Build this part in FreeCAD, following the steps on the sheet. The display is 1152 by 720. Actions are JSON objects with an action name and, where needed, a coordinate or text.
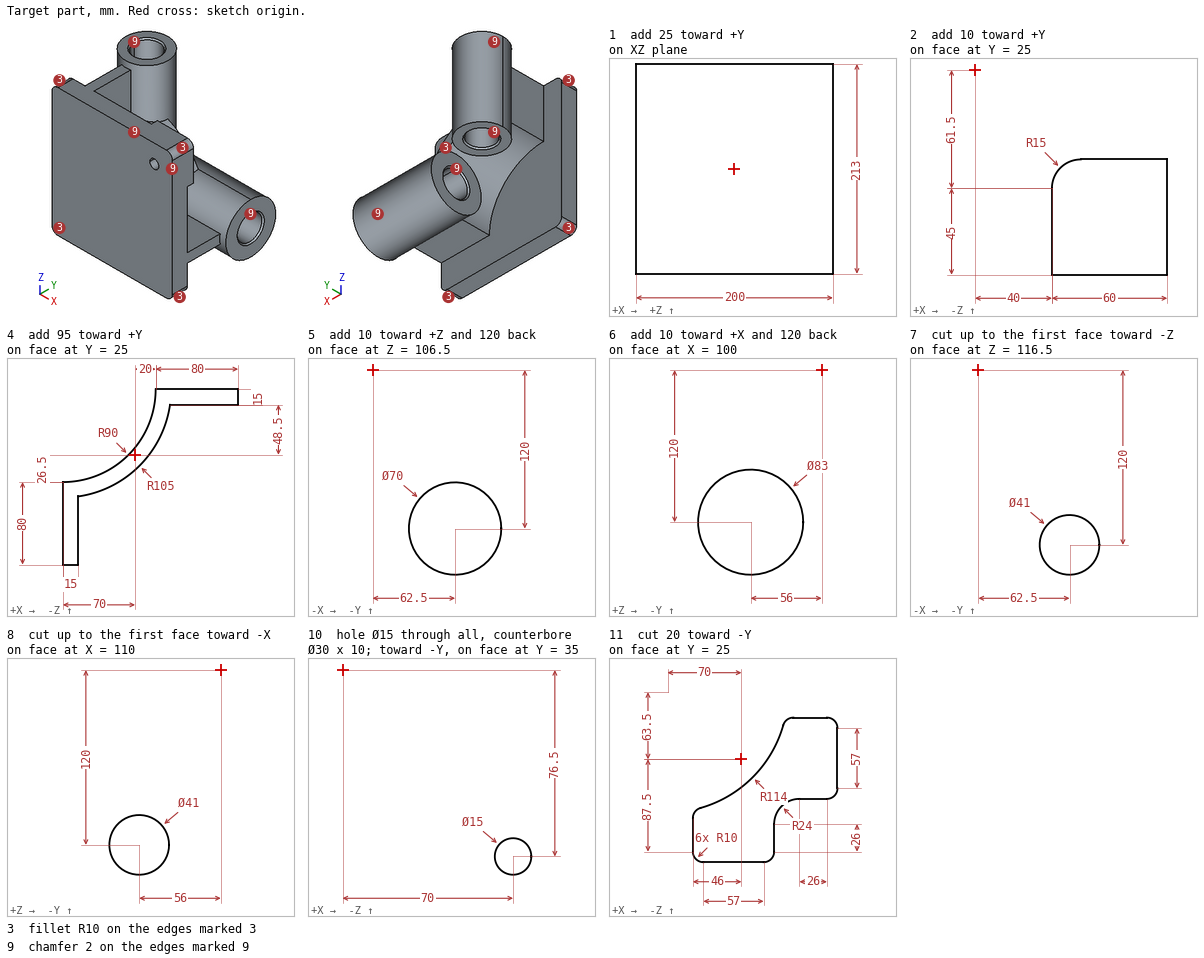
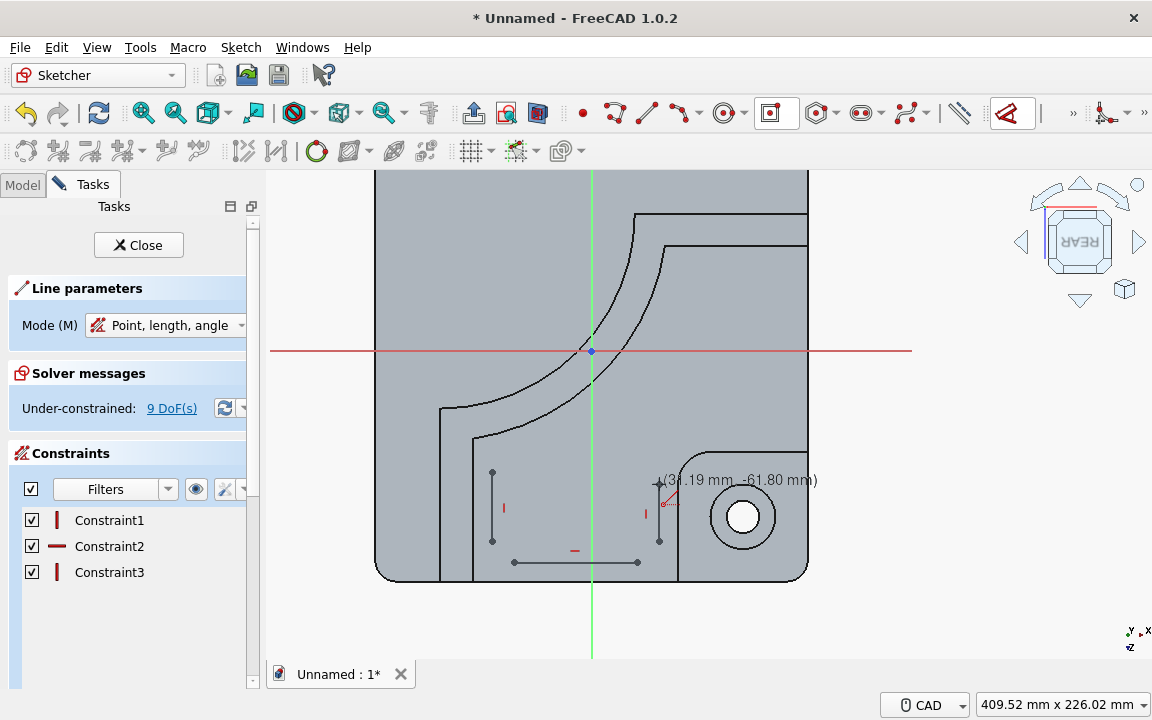
{"action": "left_click", "coordinate": [711, 432]}
{"action": "left_click", "coordinate": [767, 432]}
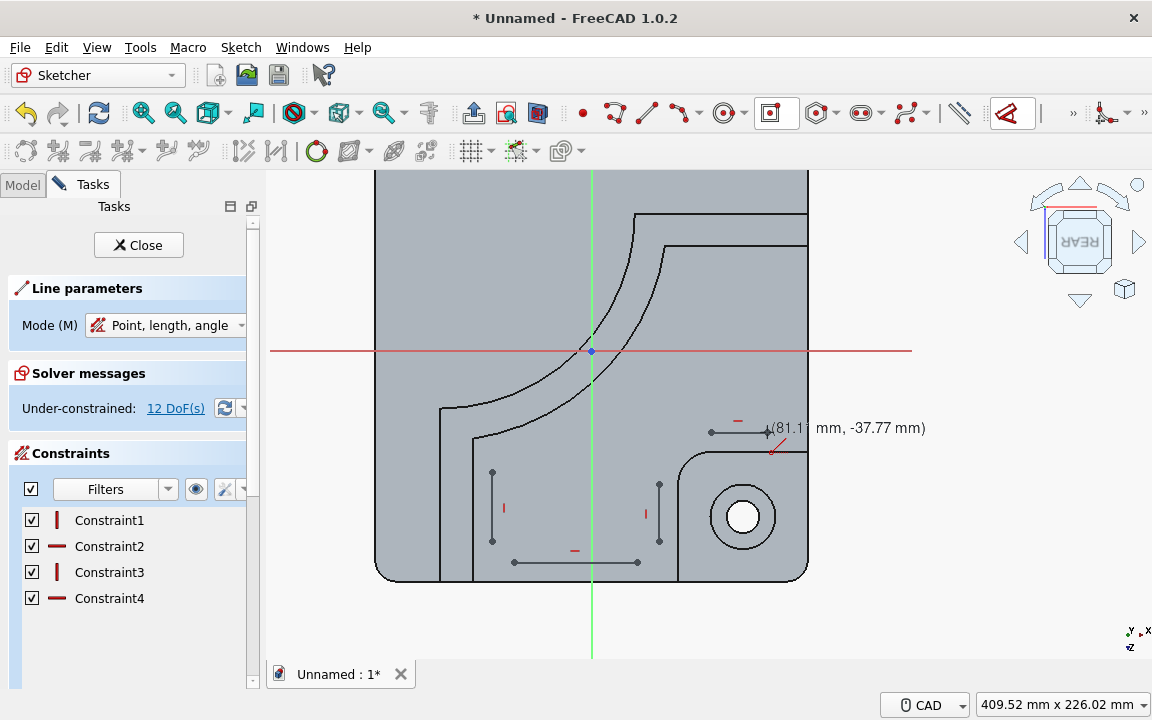
{"action": "left_click", "coordinate": [788, 411]}
{"action": "left_click", "coordinate": [788, 287]}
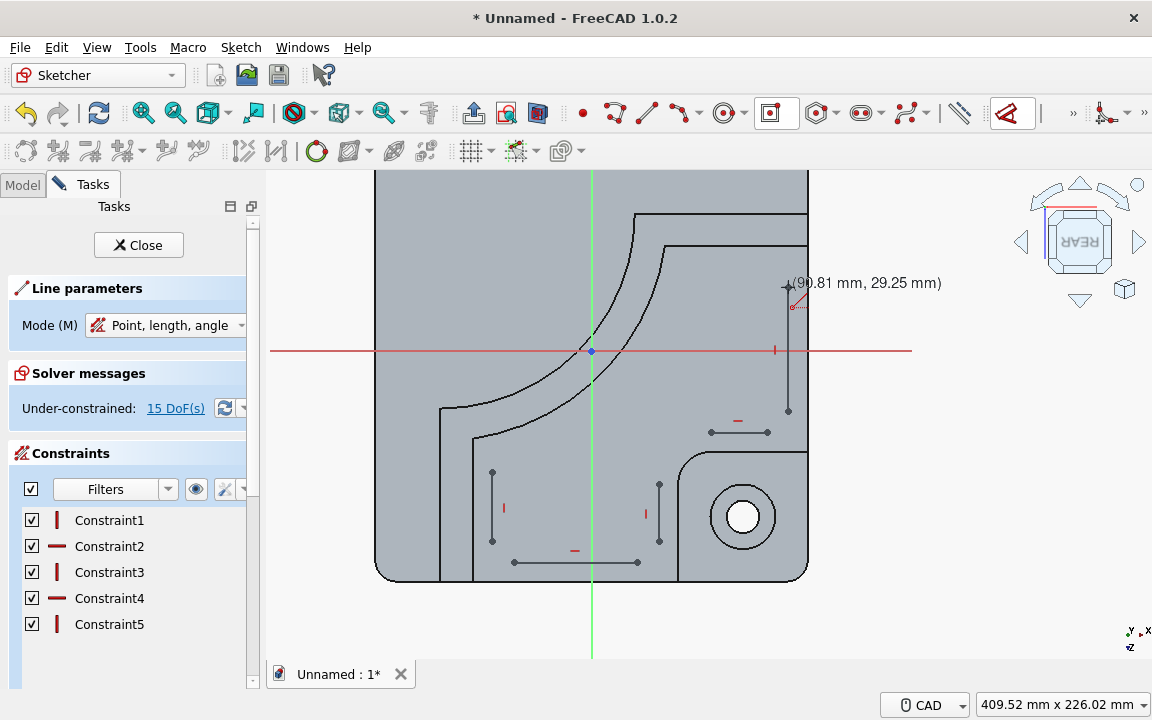
{"action": "left_click", "coordinate": [767, 266]}
{"action": "left_click", "coordinate": [698, 266]}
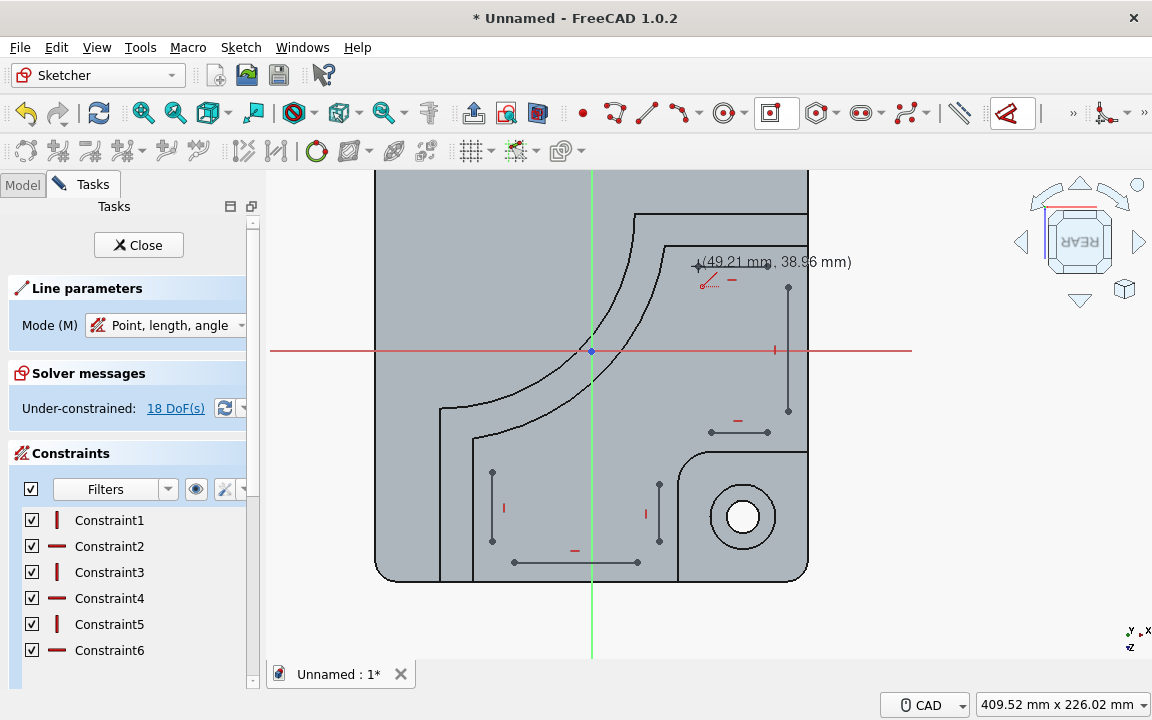
{"action": "left_click", "coordinate": [680, 114]}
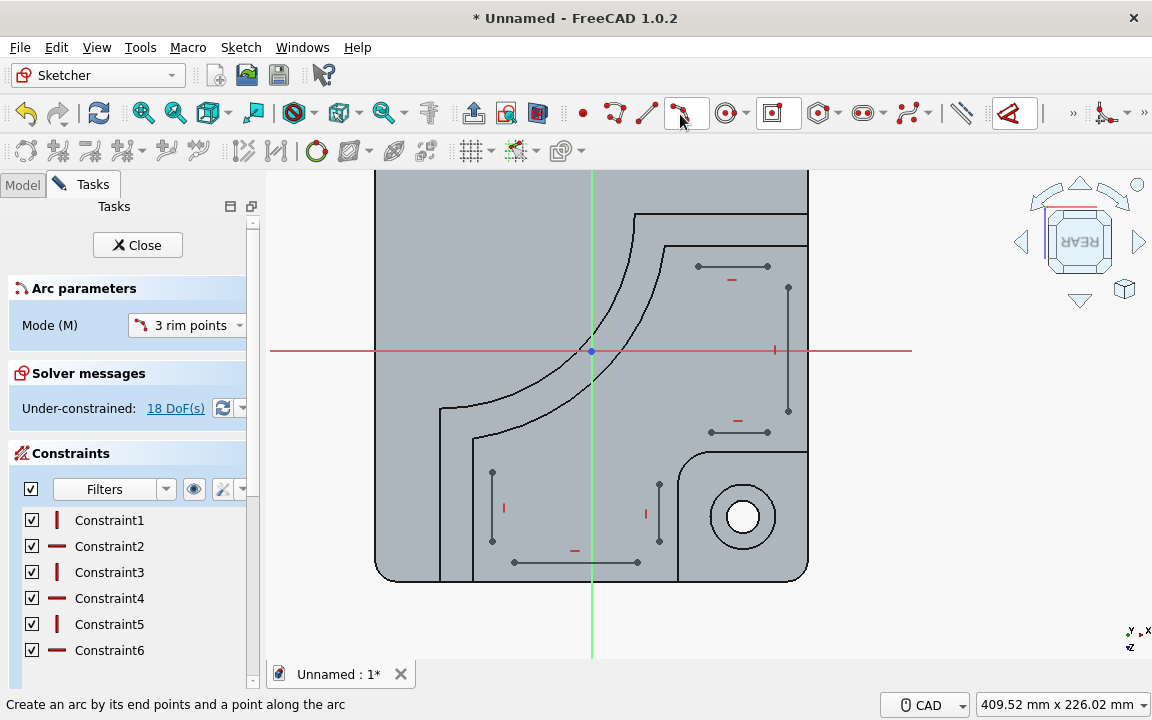
{"action": "left_click", "coordinate": [492, 542]}
{"action": "left_click", "coordinate": [514, 563]}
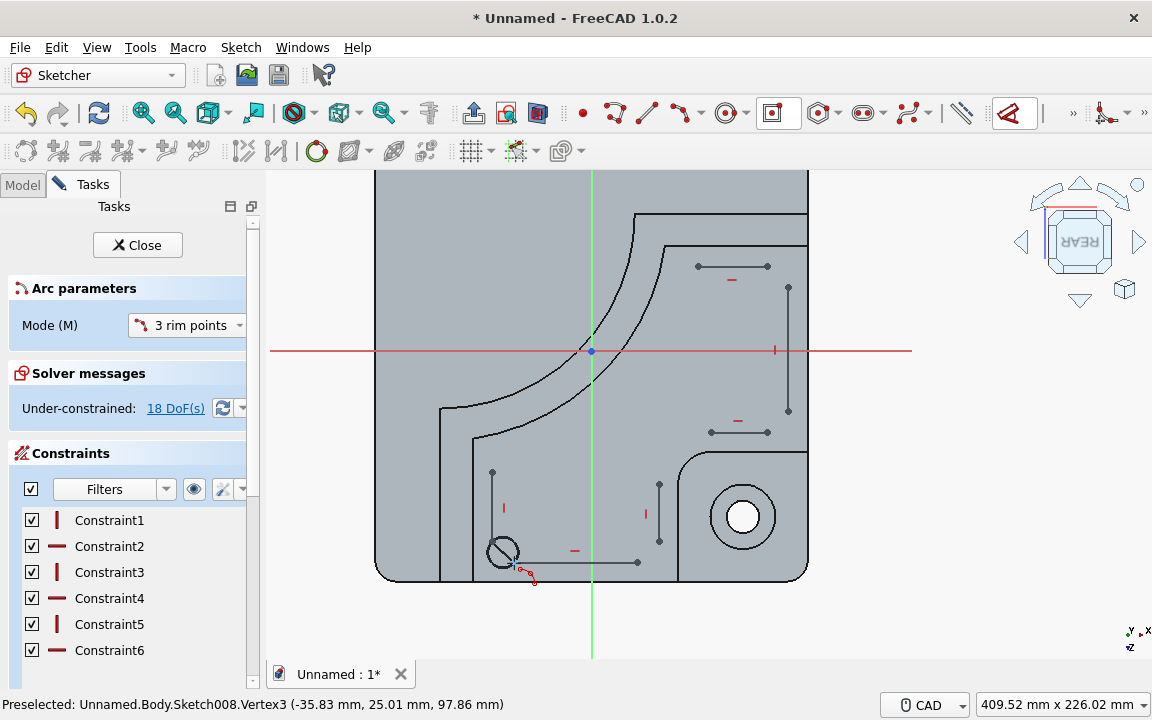
{"action": "scroll", "coordinate": [498, 556], "scroll_direction": "up", "scroll_amount": 5}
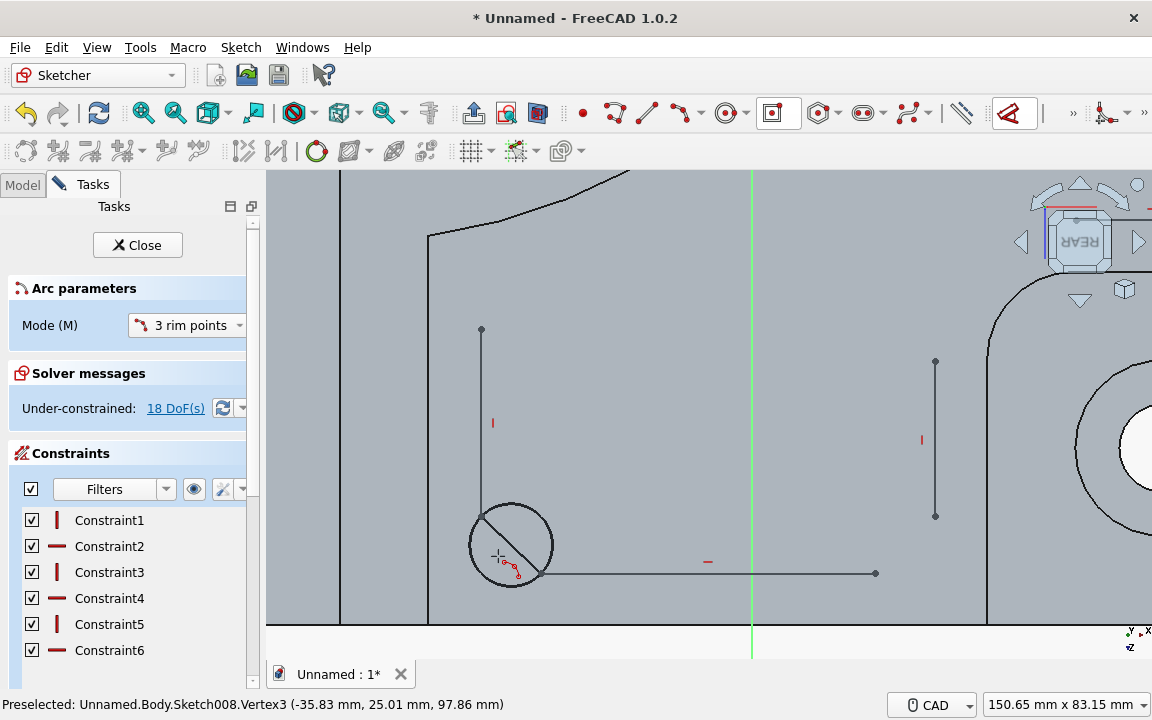
{"action": "left_click", "coordinate": [498, 554]}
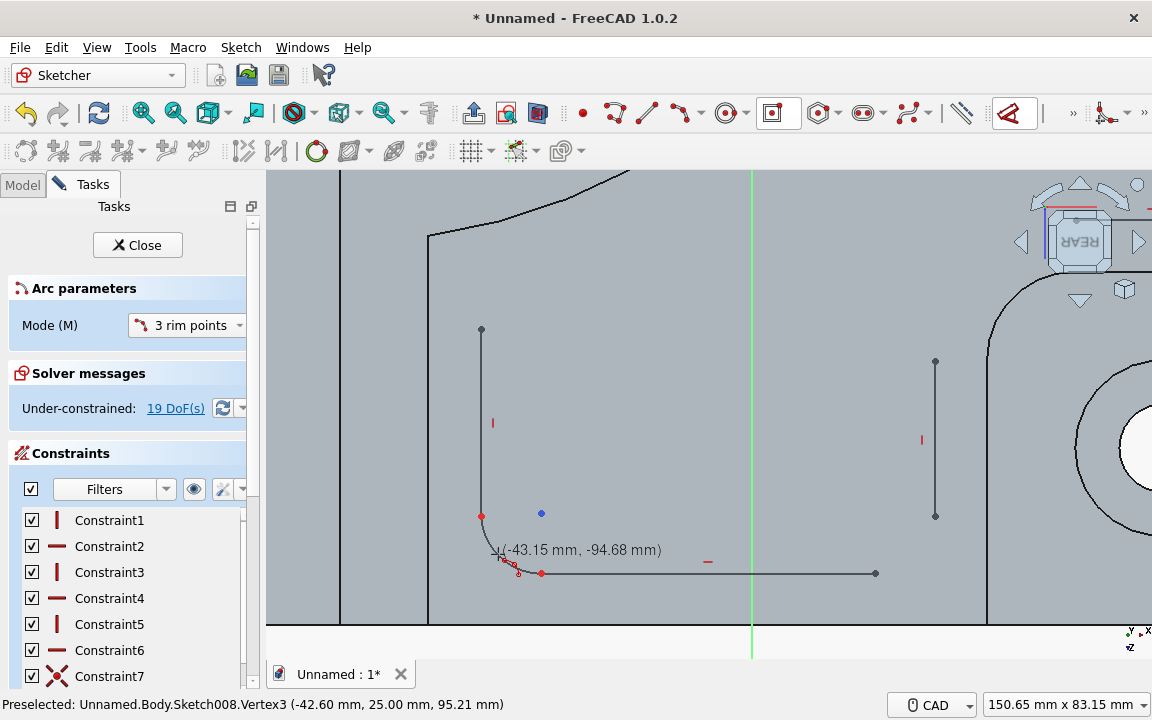
{"action": "left_click", "coordinate": [875, 574]}
{"action": "left_click", "coordinate": [935, 517]}
{"action": "left_click", "coordinate": [917, 554]}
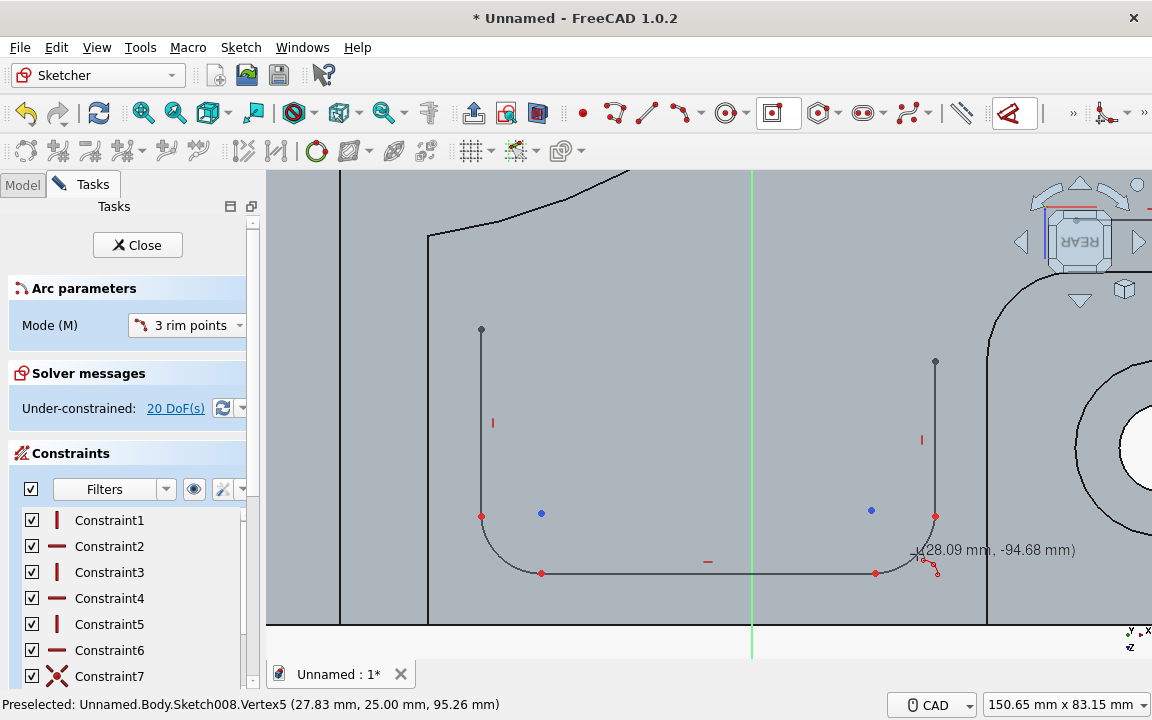
{"action": "left_click", "coordinate": [935, 362]}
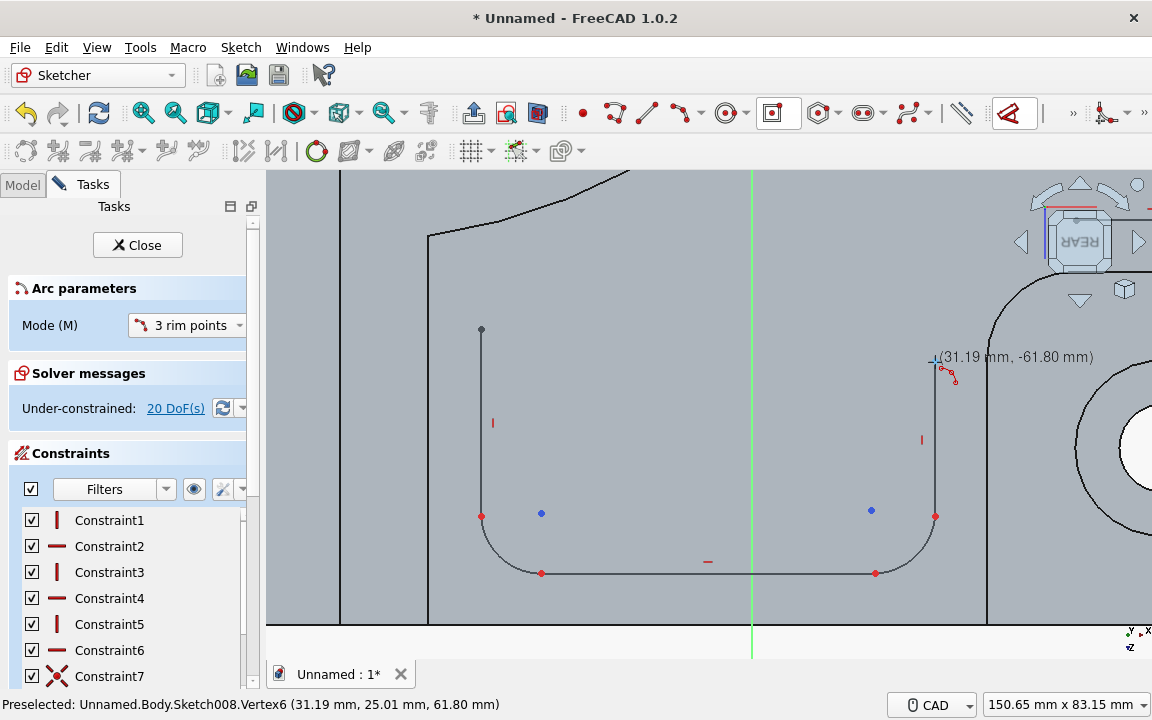
{"action": "scroll", "coordinate": [499, 558], "scroll_direction": "down", "scroll_amount": 5}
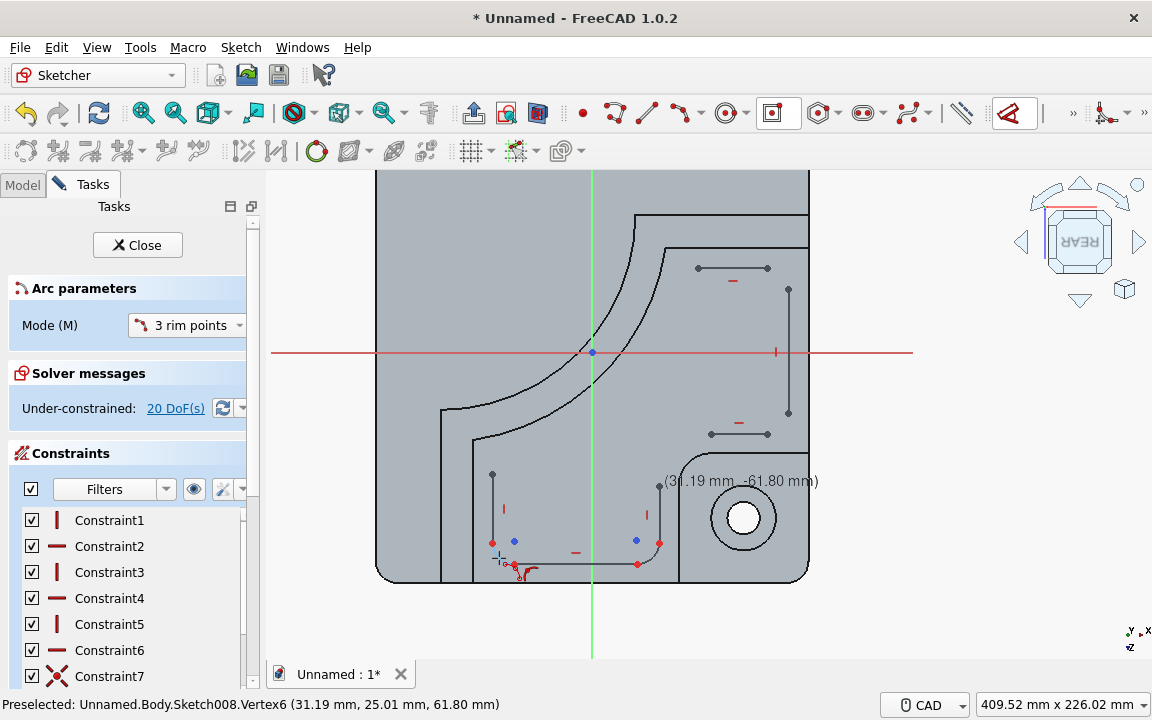
{"action": "left_click", "coordinate": [712, 434]}
{"action": "left_click", "coordinate": [674, 449]}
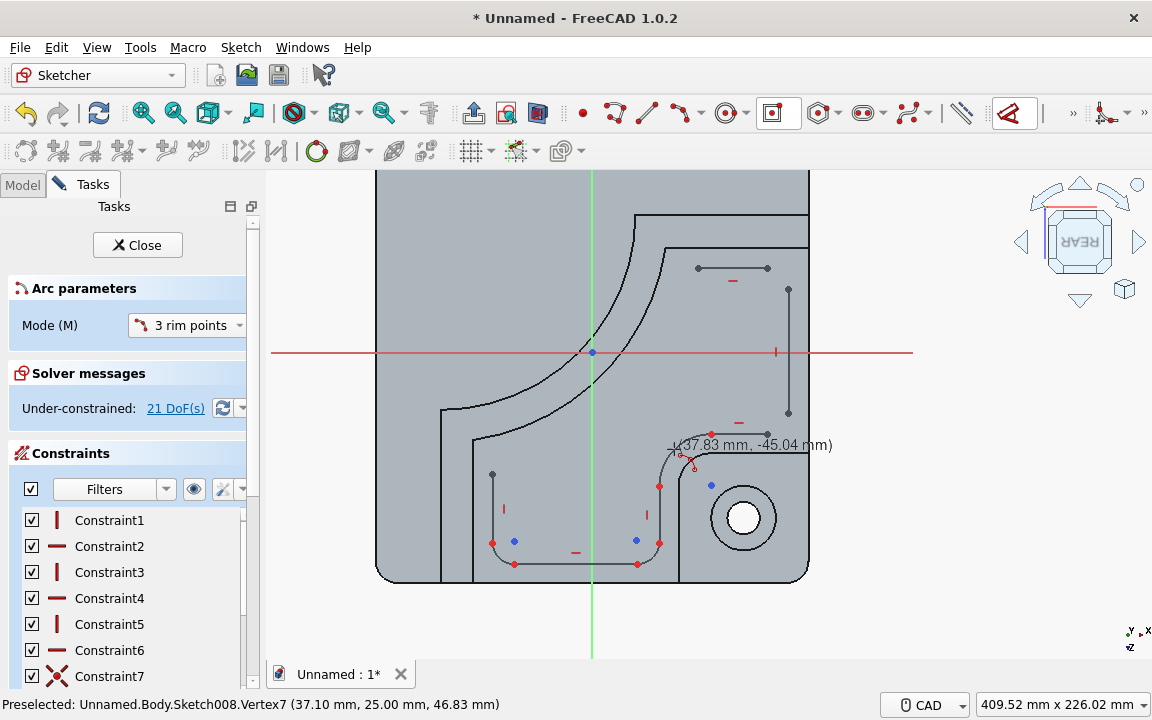
{"action": "left_click", "coordinate": [768, 434]}
{"action": "left_click", "coordinate": [789, 413]}